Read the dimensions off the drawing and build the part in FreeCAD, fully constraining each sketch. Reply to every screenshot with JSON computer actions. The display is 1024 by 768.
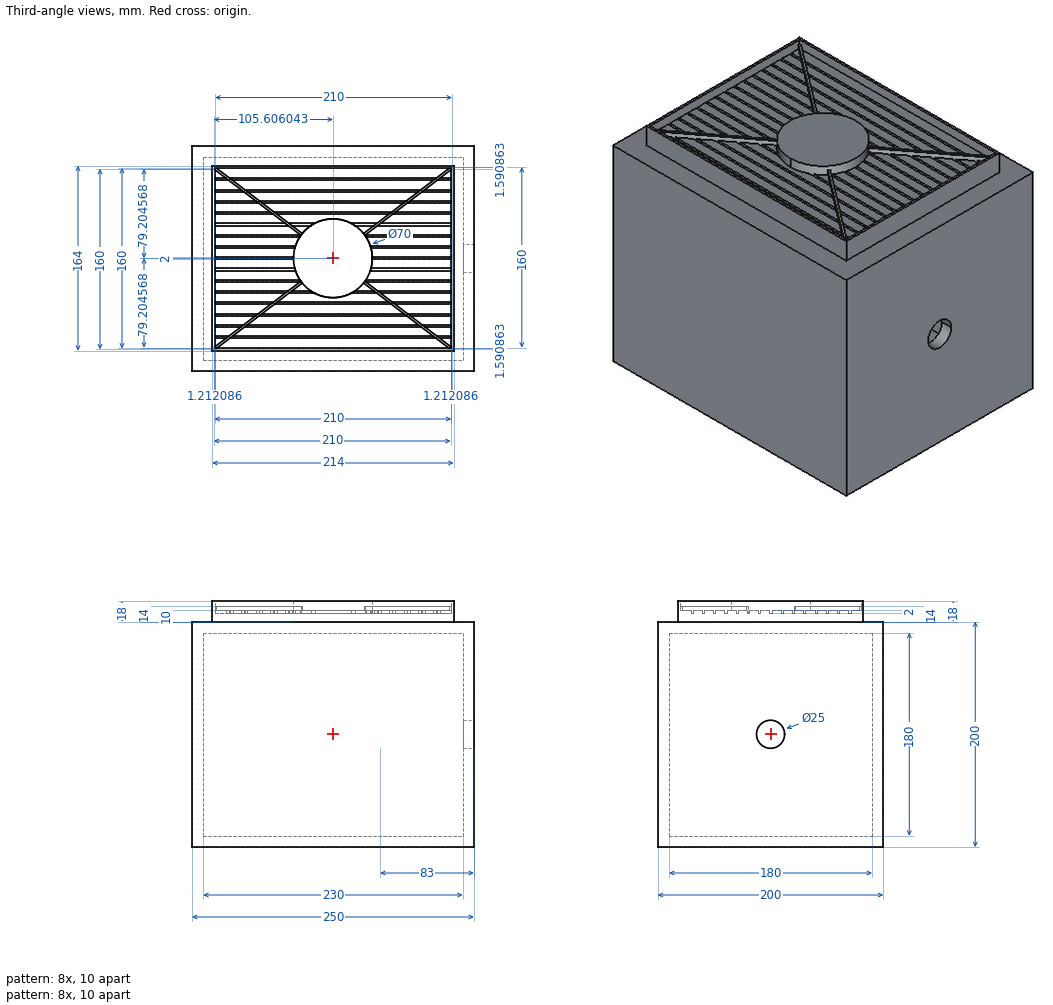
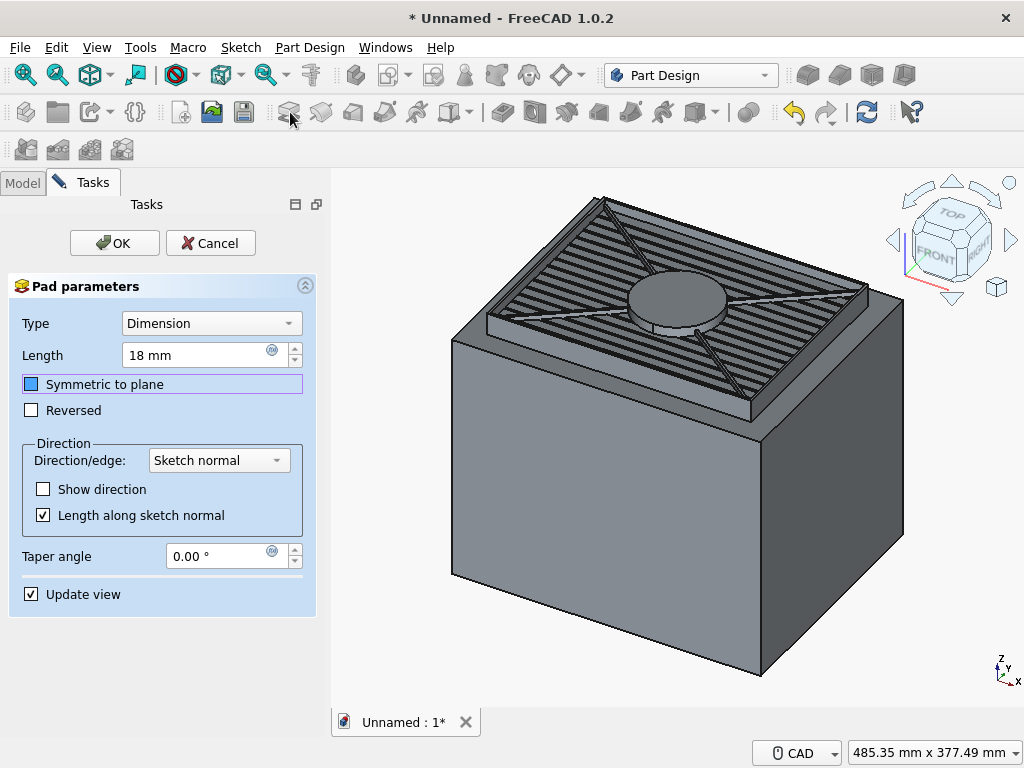
{"action": "left_click", "coordinate": [115, 243]}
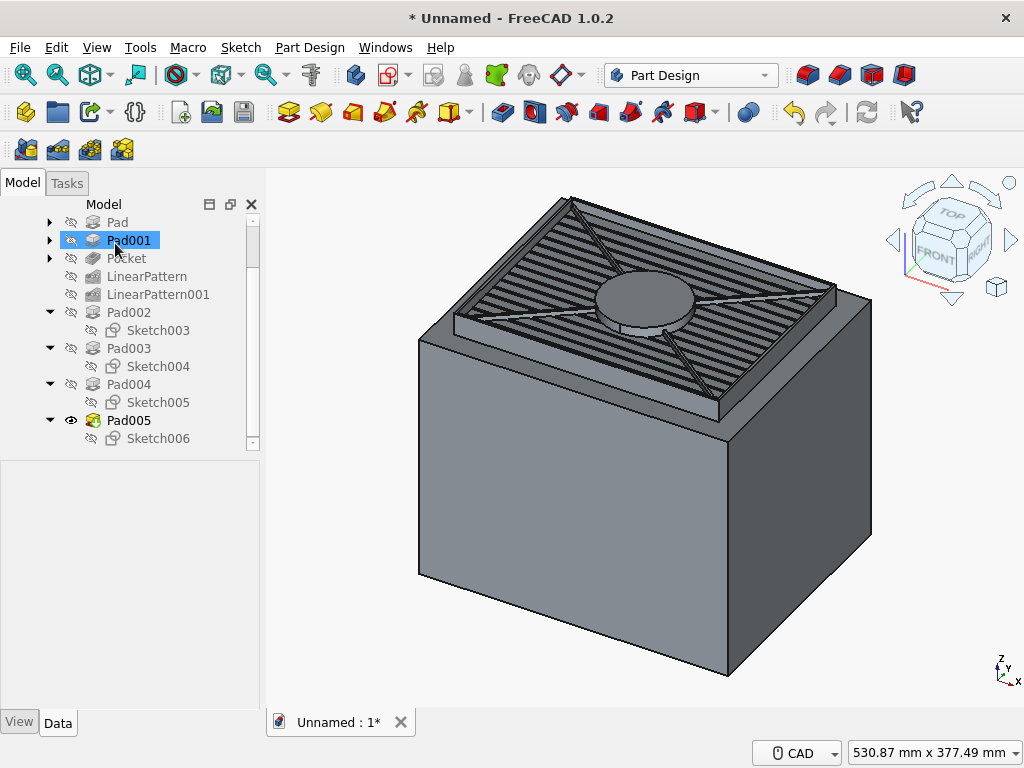
{"action": "scroll", "coordinate": [140, 326], "scroll_direction": "down", "scroll_amount": 3}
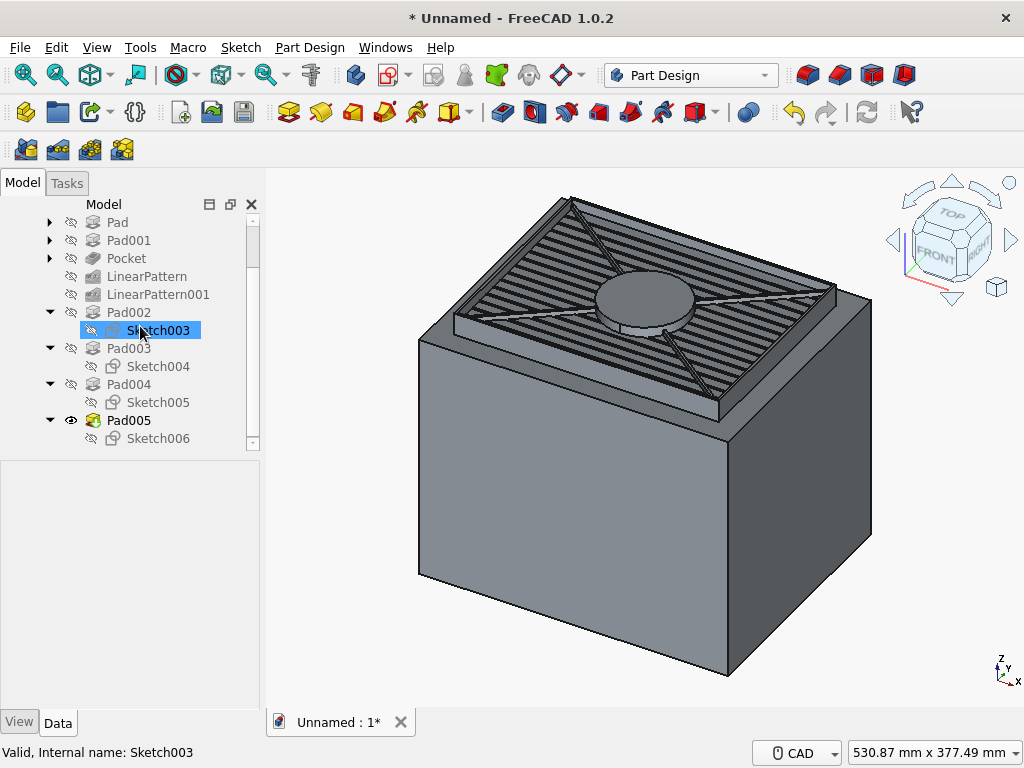
{"action": "scroll", "coordinate": [140, 326], "scroll_direction": "up", "scroll_amount": 15}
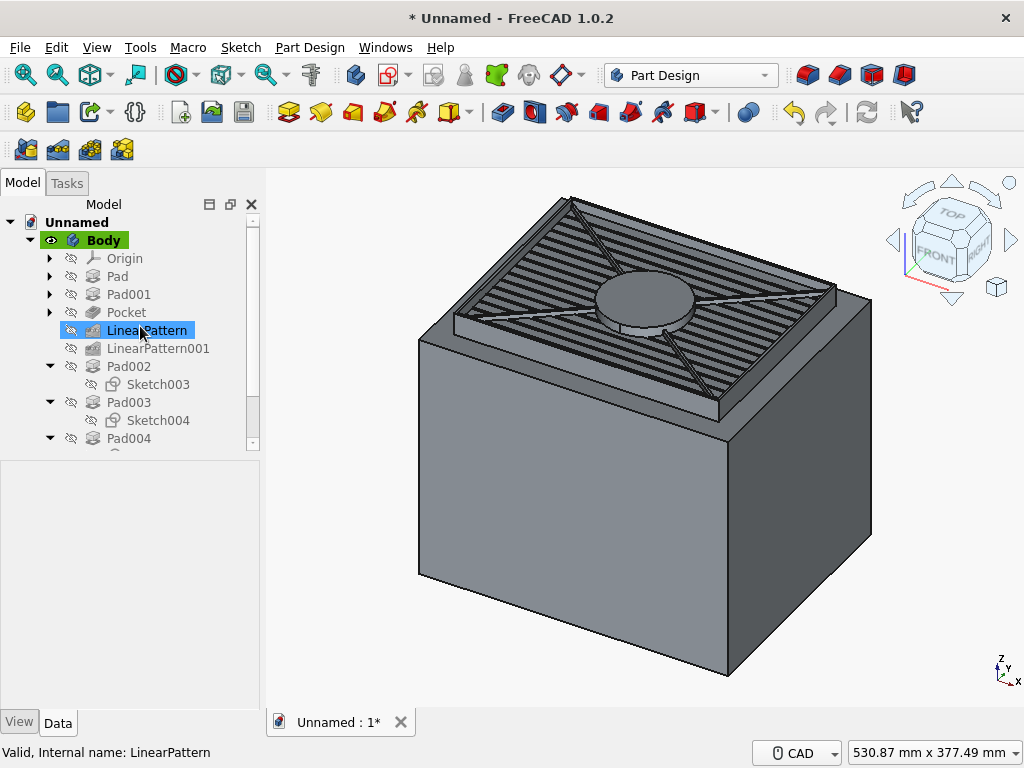
{"action": "left_click", "coordinate": [50, 258]}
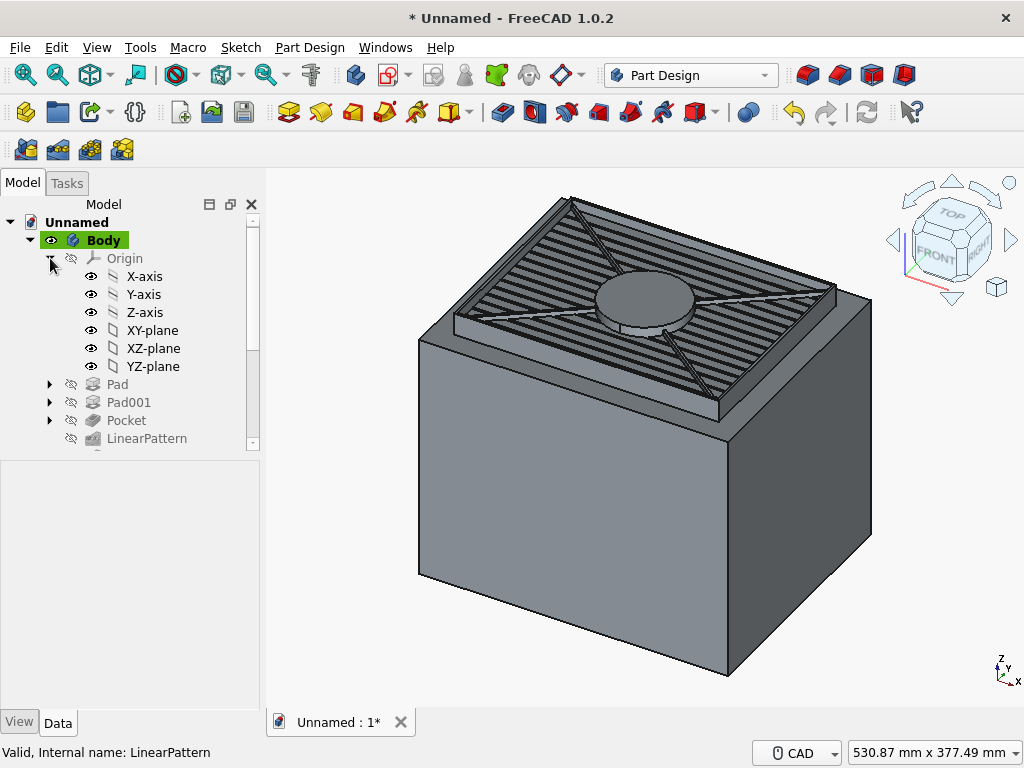
{"action": "left_click", "coordinate": [136, 366]}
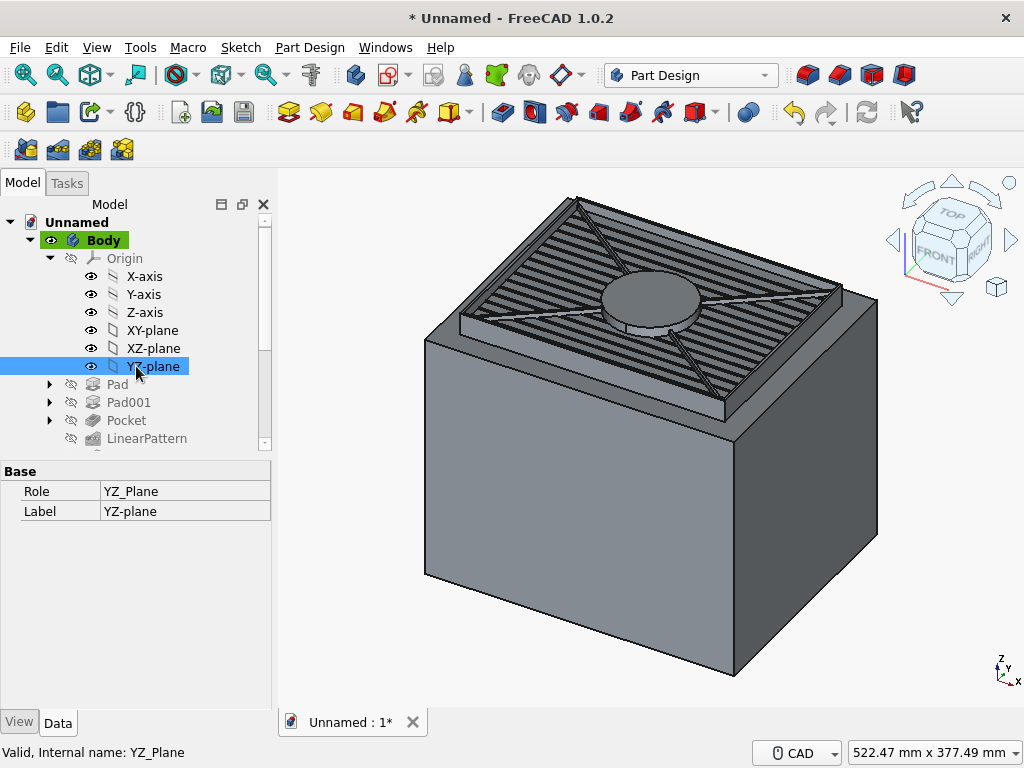
{"action": "left_click", "coordinate": [562, 76]}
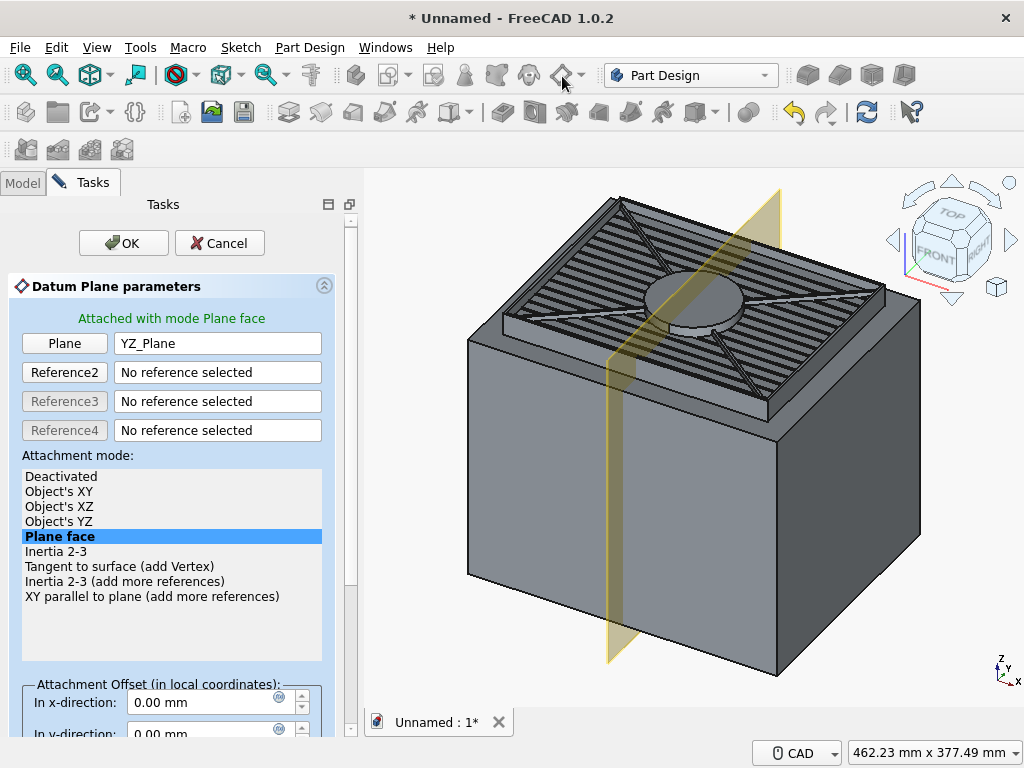
{"action": "scroll", "coordinate": [351, 475], "scroll_direction": "down", "scroll_amount": 2}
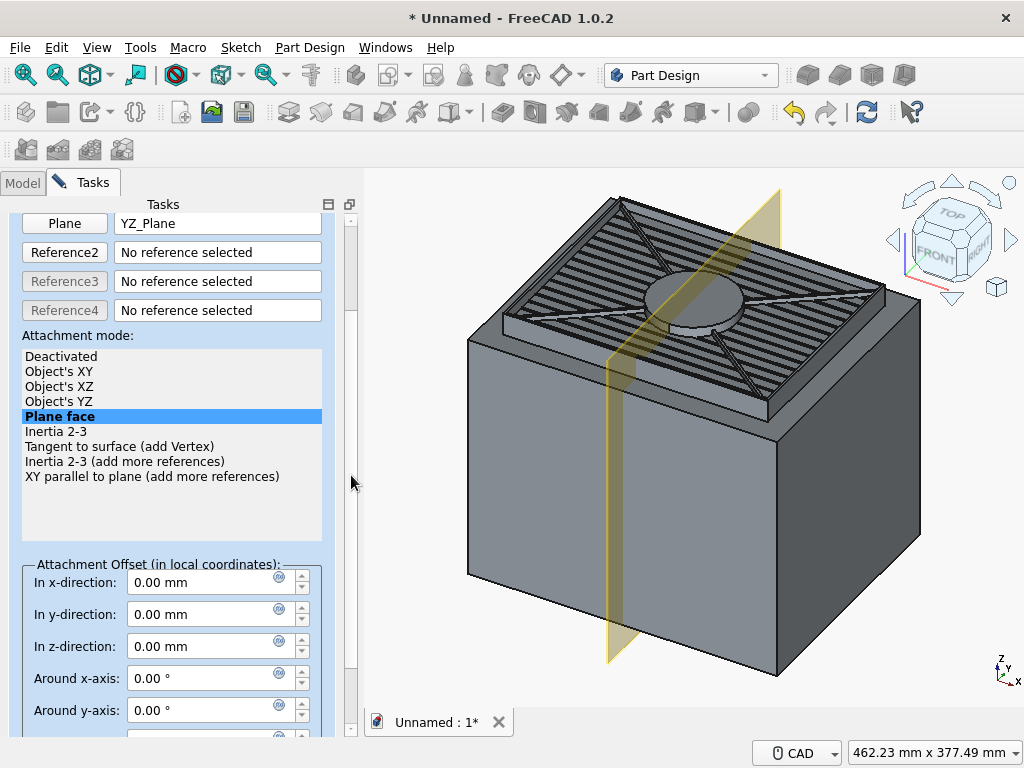
{"action": "triple_click", "coordinate": [210, 646]}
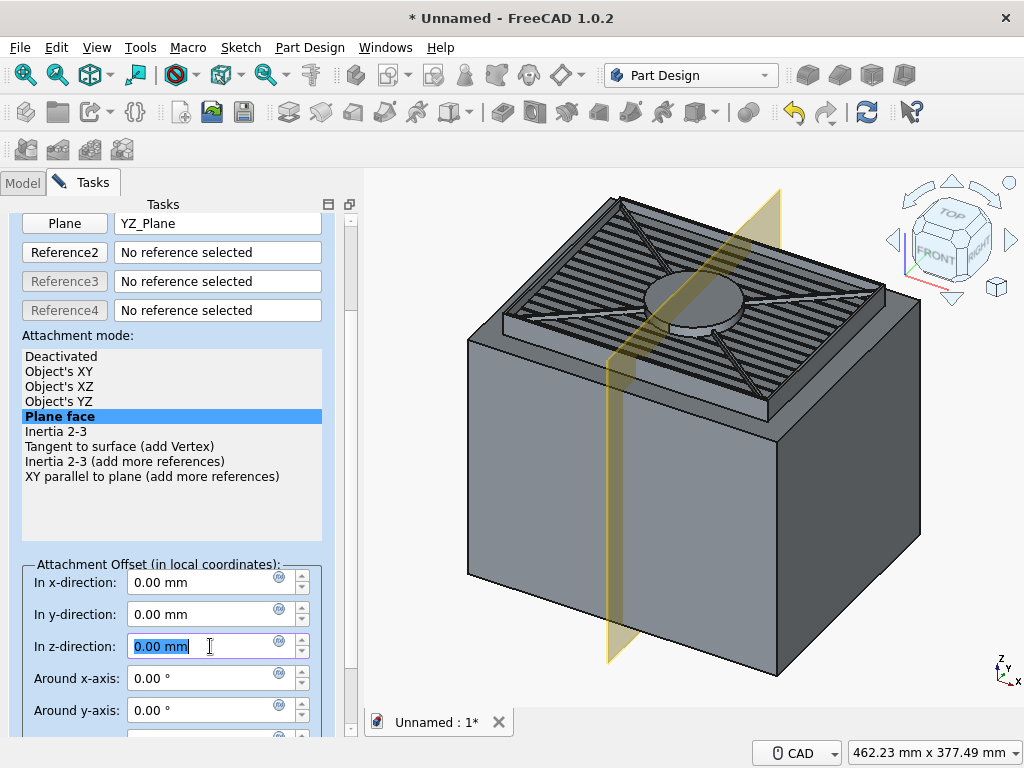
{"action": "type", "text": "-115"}
{"action": "key", "text": "Tab"}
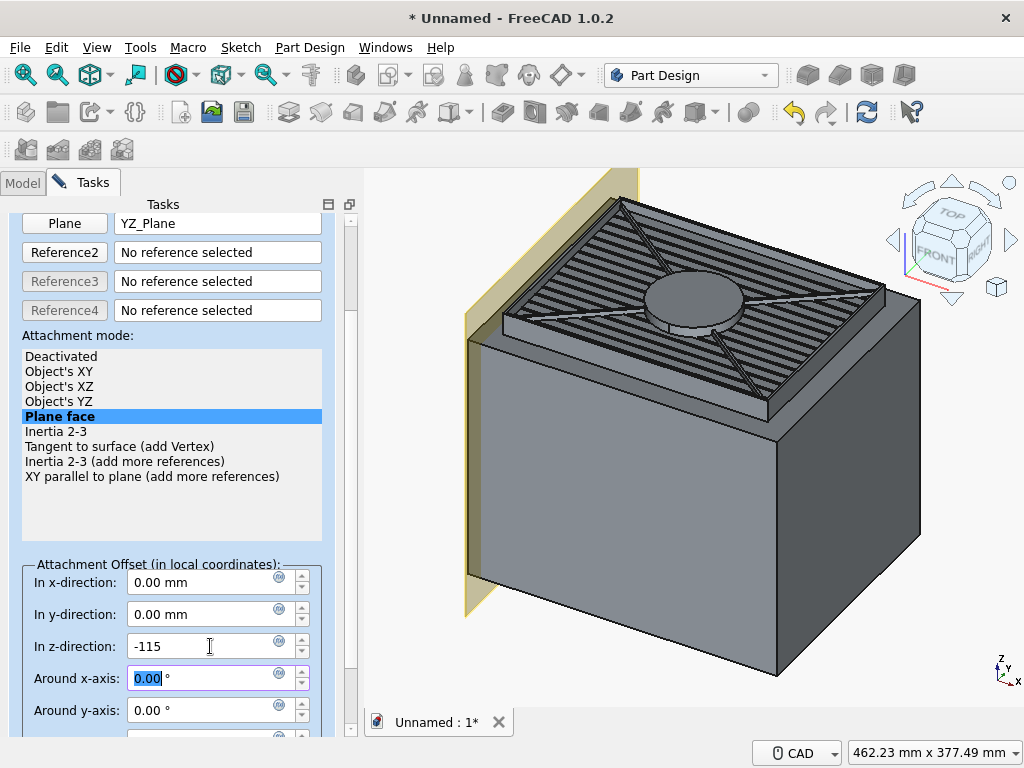
{"action": "scroll", "coordinate": [351, 475], "scroll_direction": "up", "scroll_amount": 3}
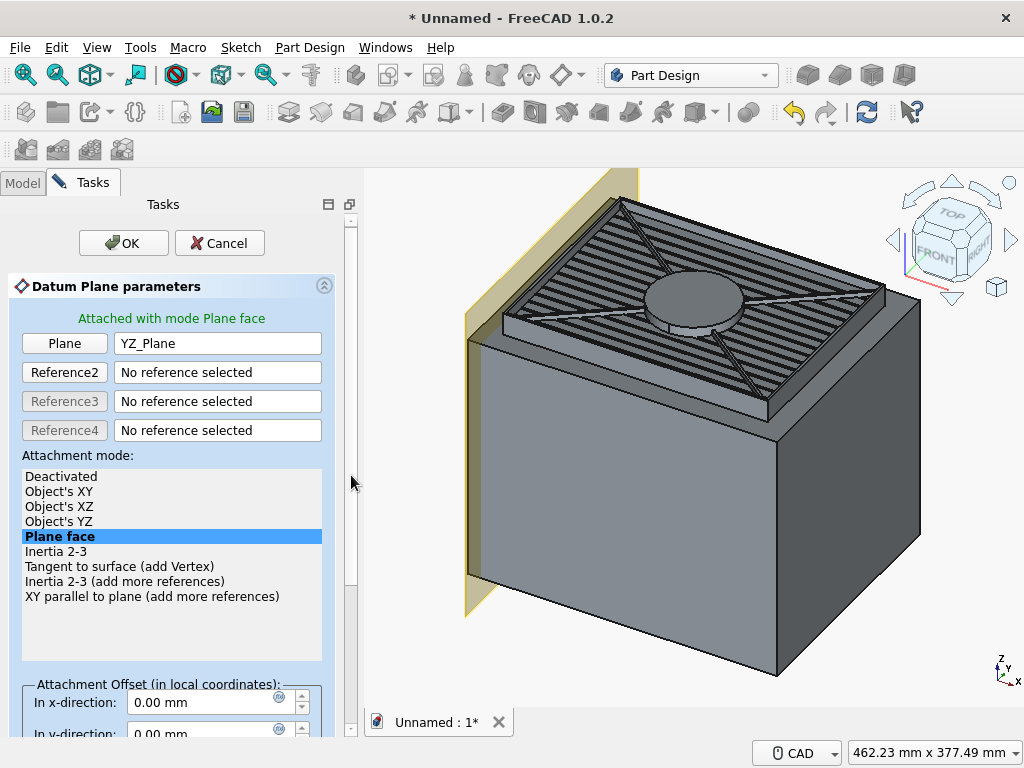
{"action": "left_click", "coordinate": [124, 243]}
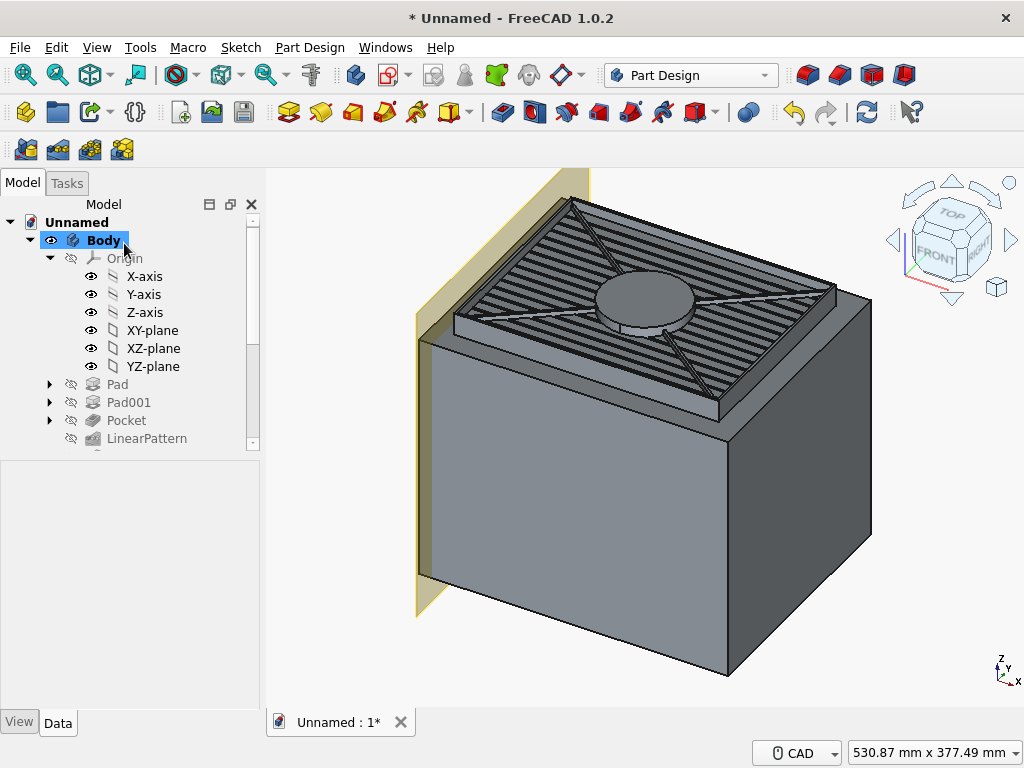
{"action": "scroll", "coordinate": [100, 326], "scroll_direction": "down", "scroll_amount": 3}